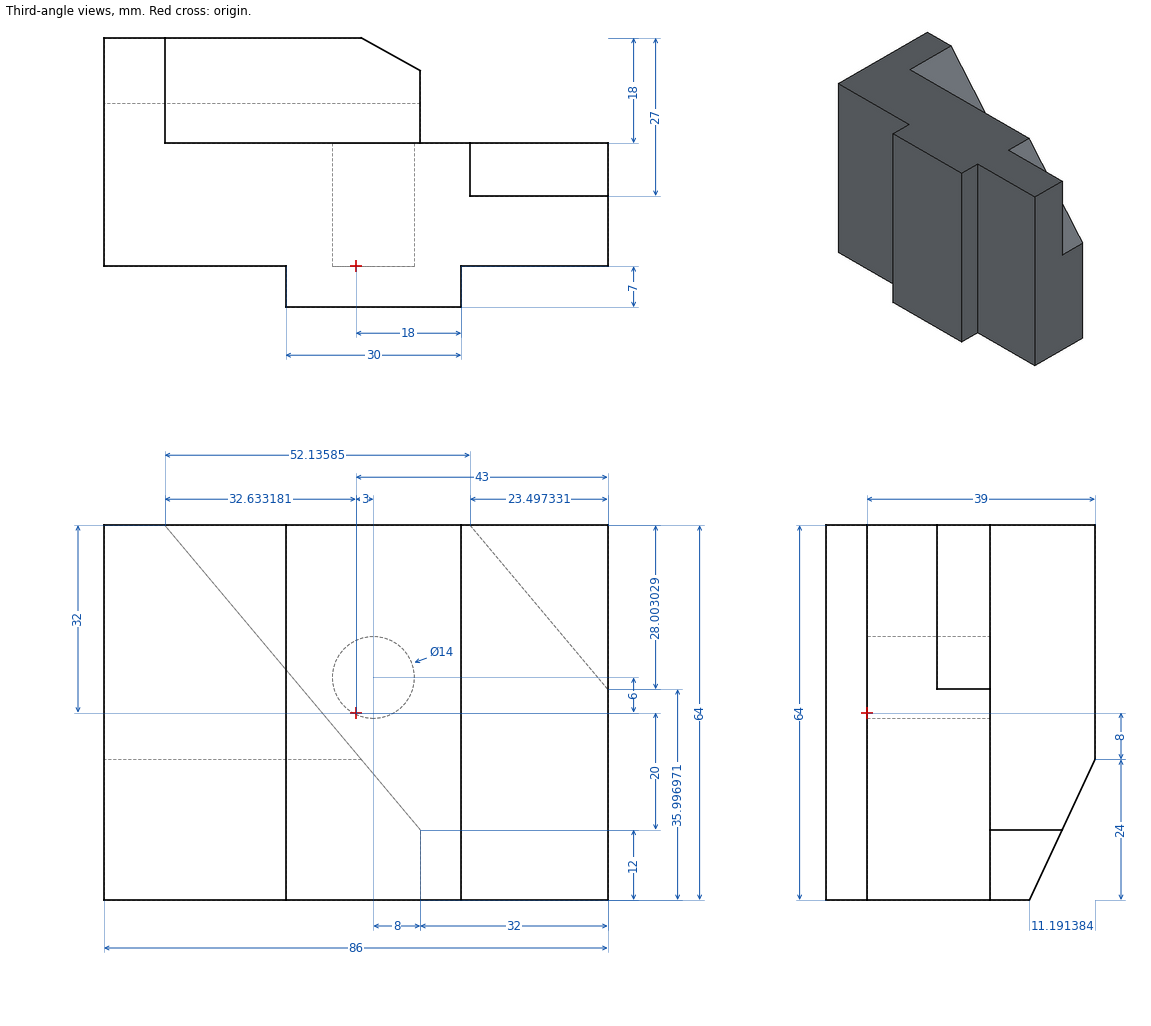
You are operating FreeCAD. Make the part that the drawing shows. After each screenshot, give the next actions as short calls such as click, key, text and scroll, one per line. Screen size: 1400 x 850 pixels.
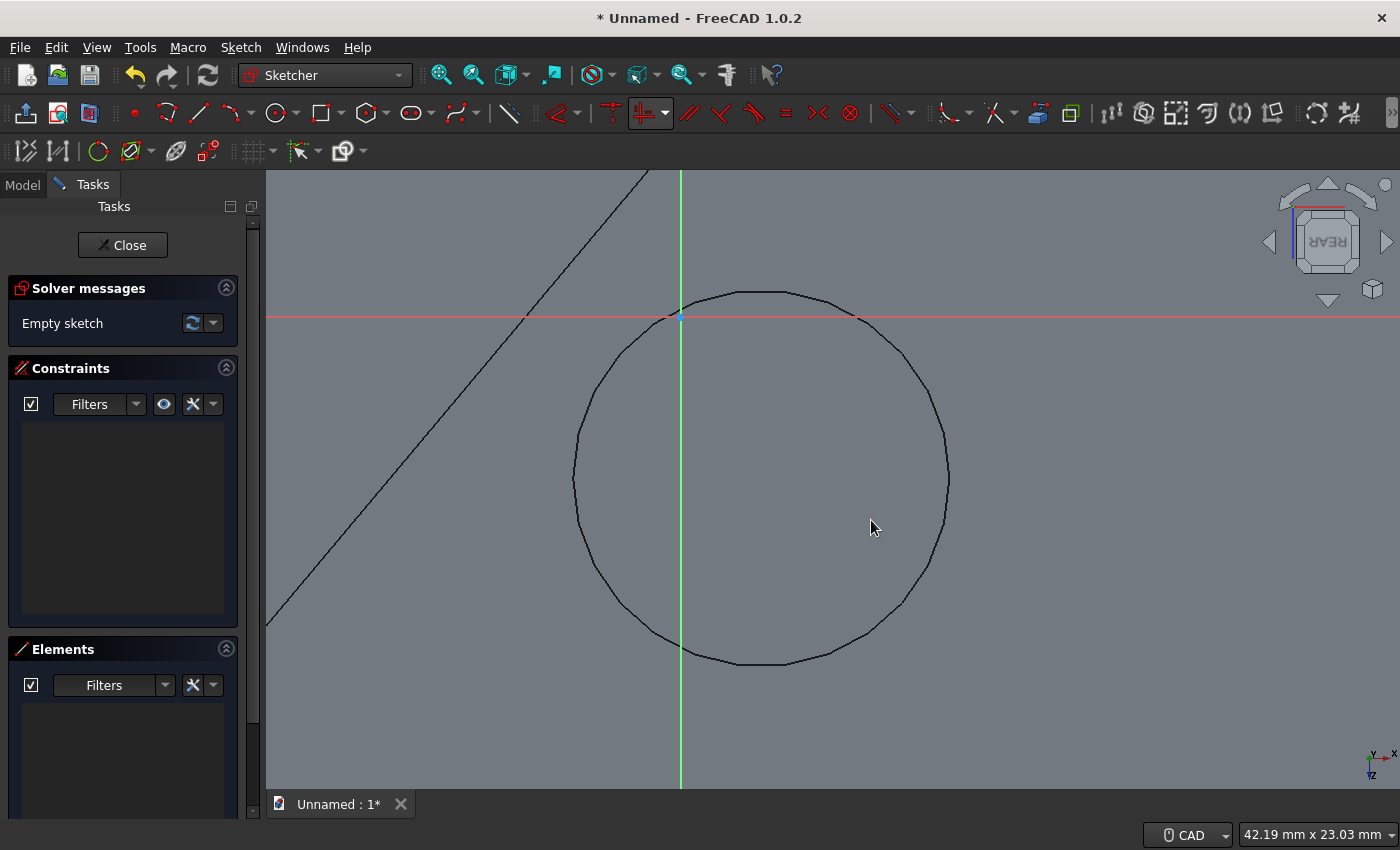
key(g)
key(c)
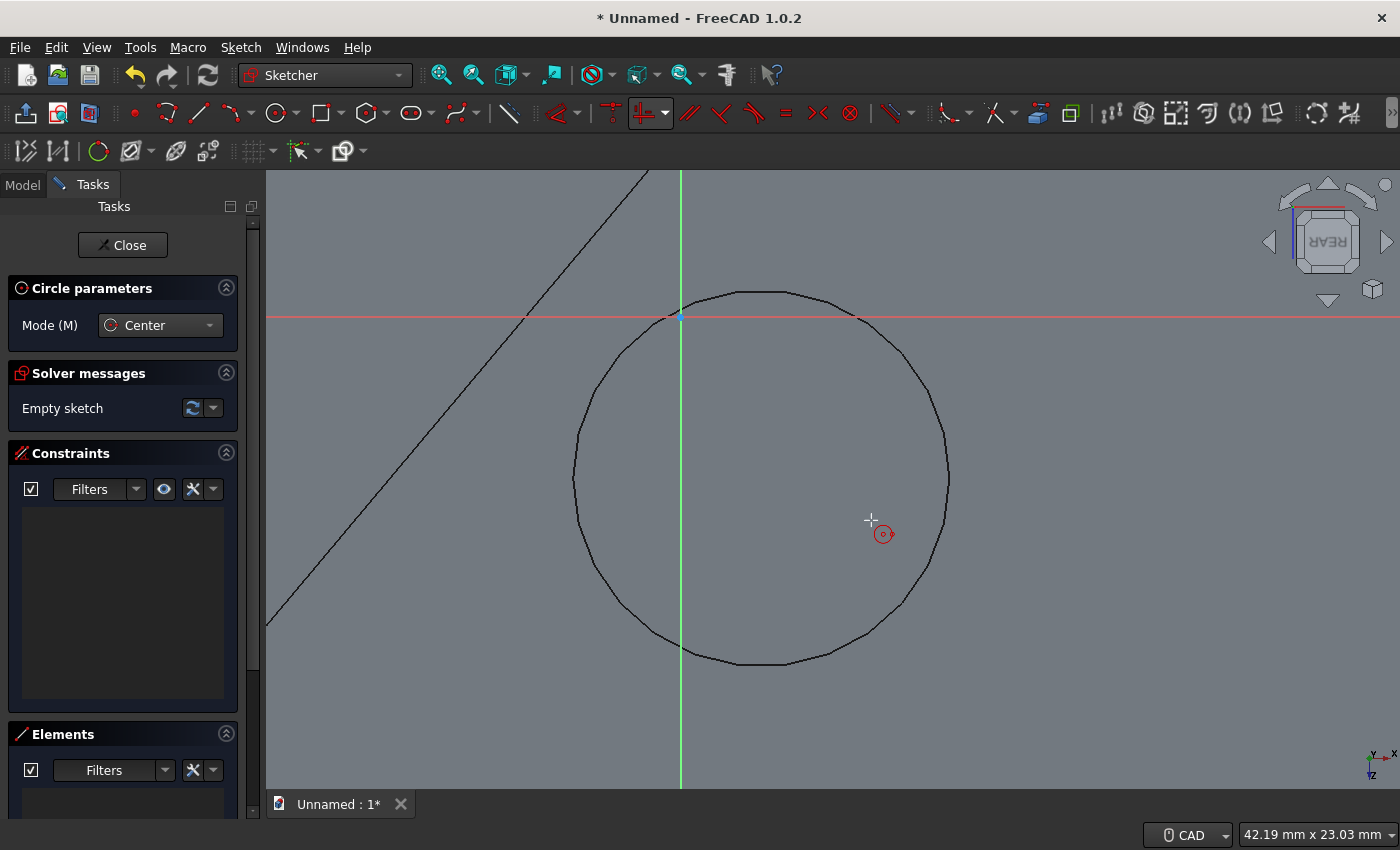
click(761, 478)
move(894, 345)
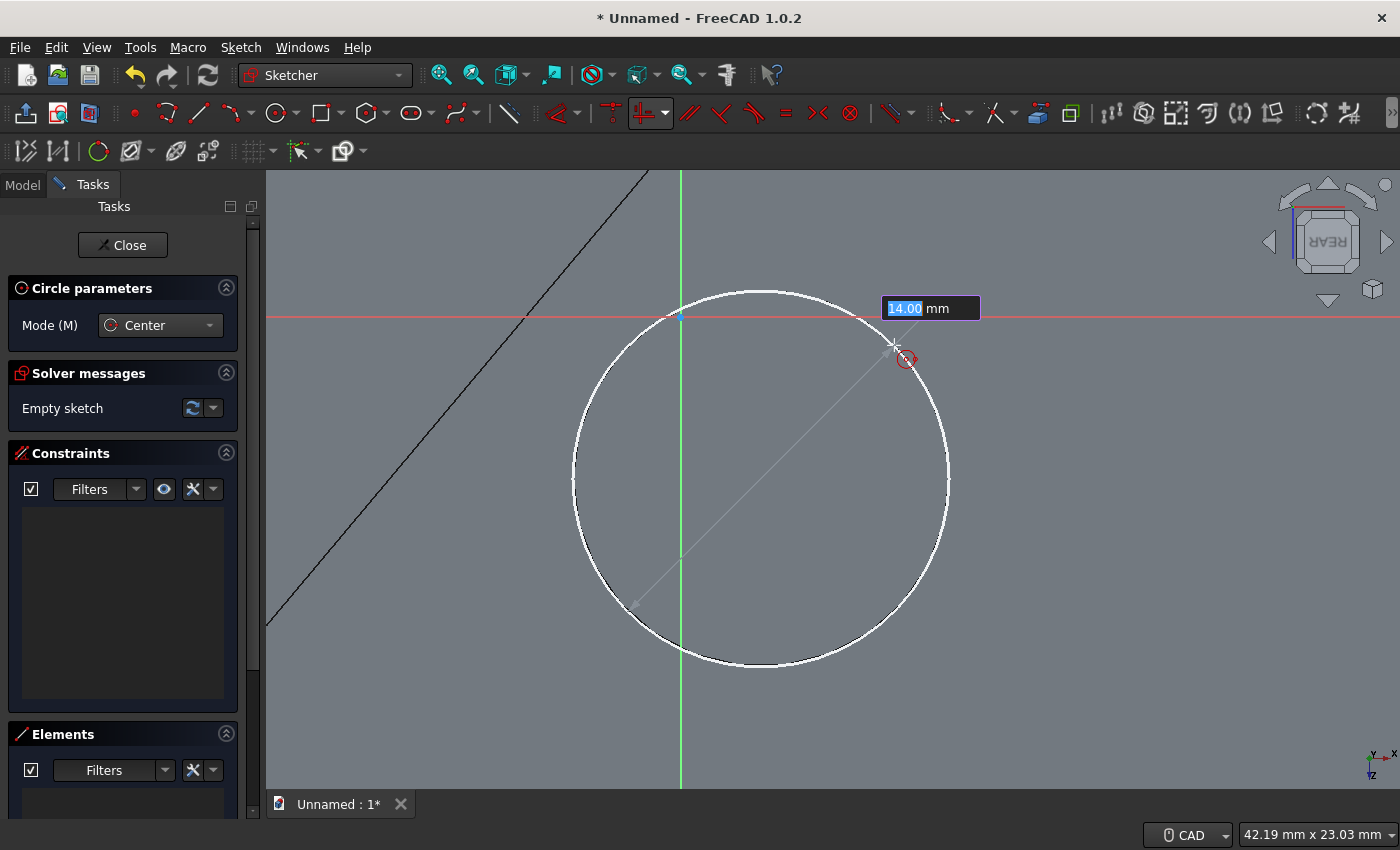
text(14)
key(Return)
key(Escape)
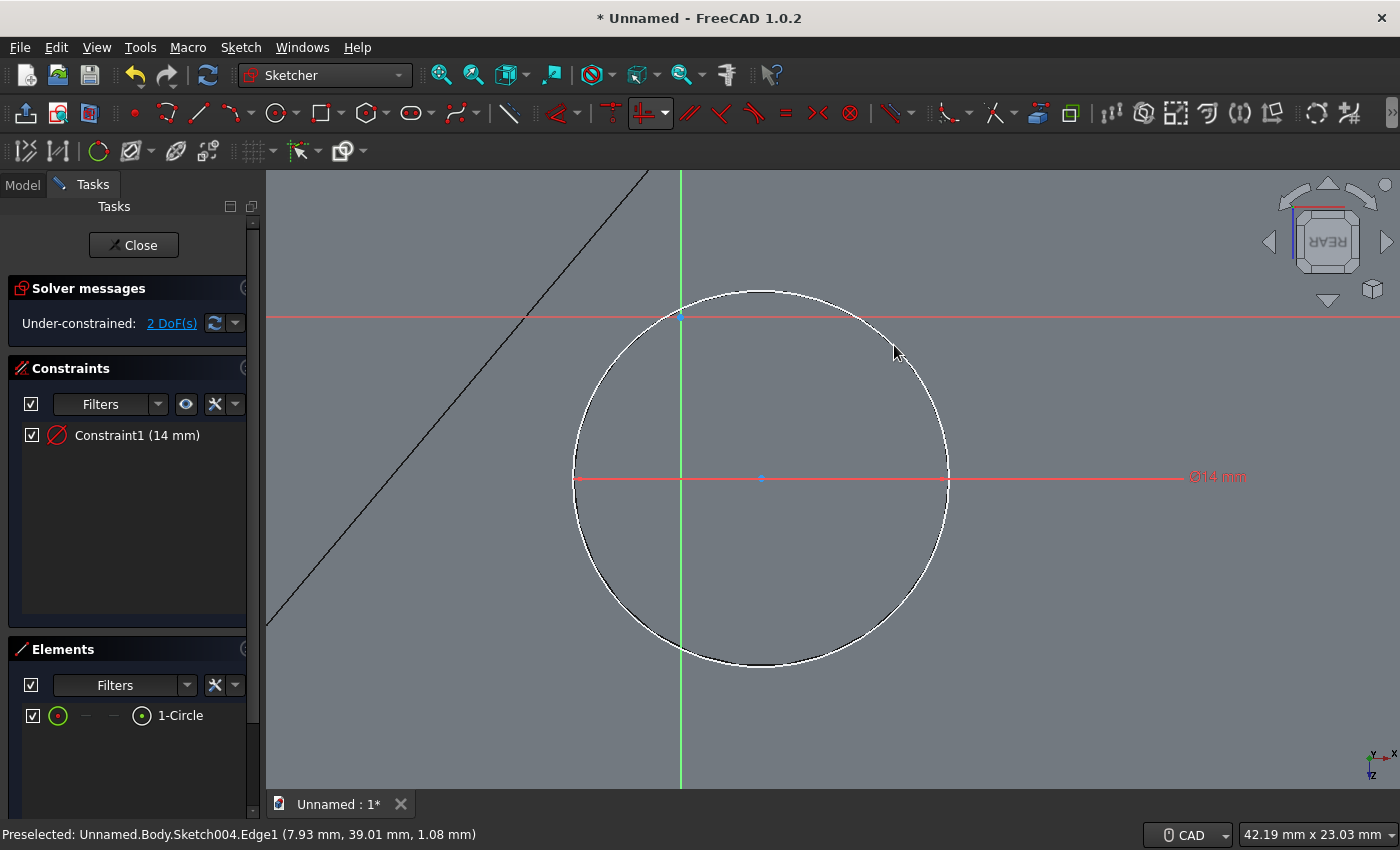
key(d)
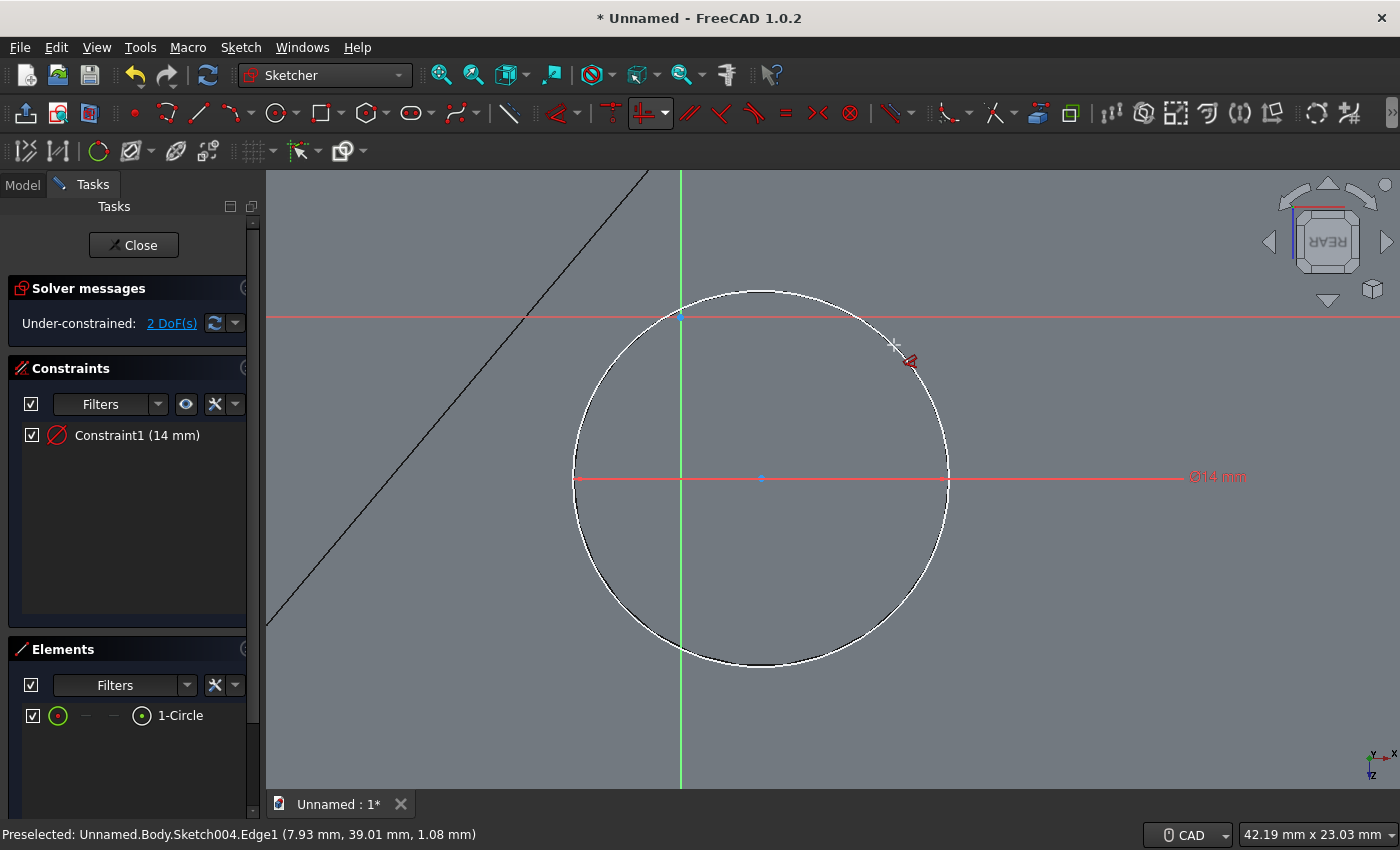
click(761, 479)
click(702, 283)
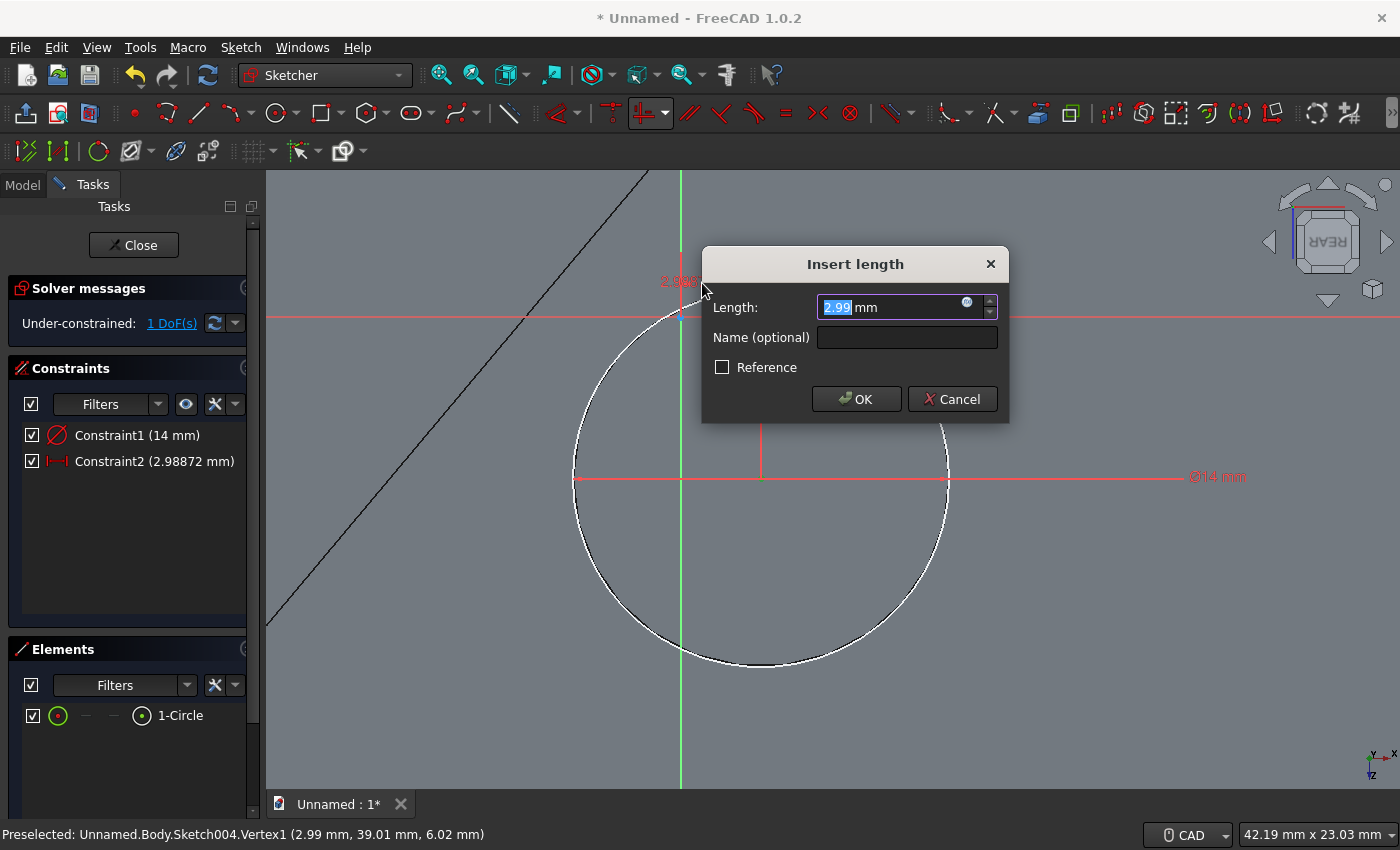
text(3)
key(Return)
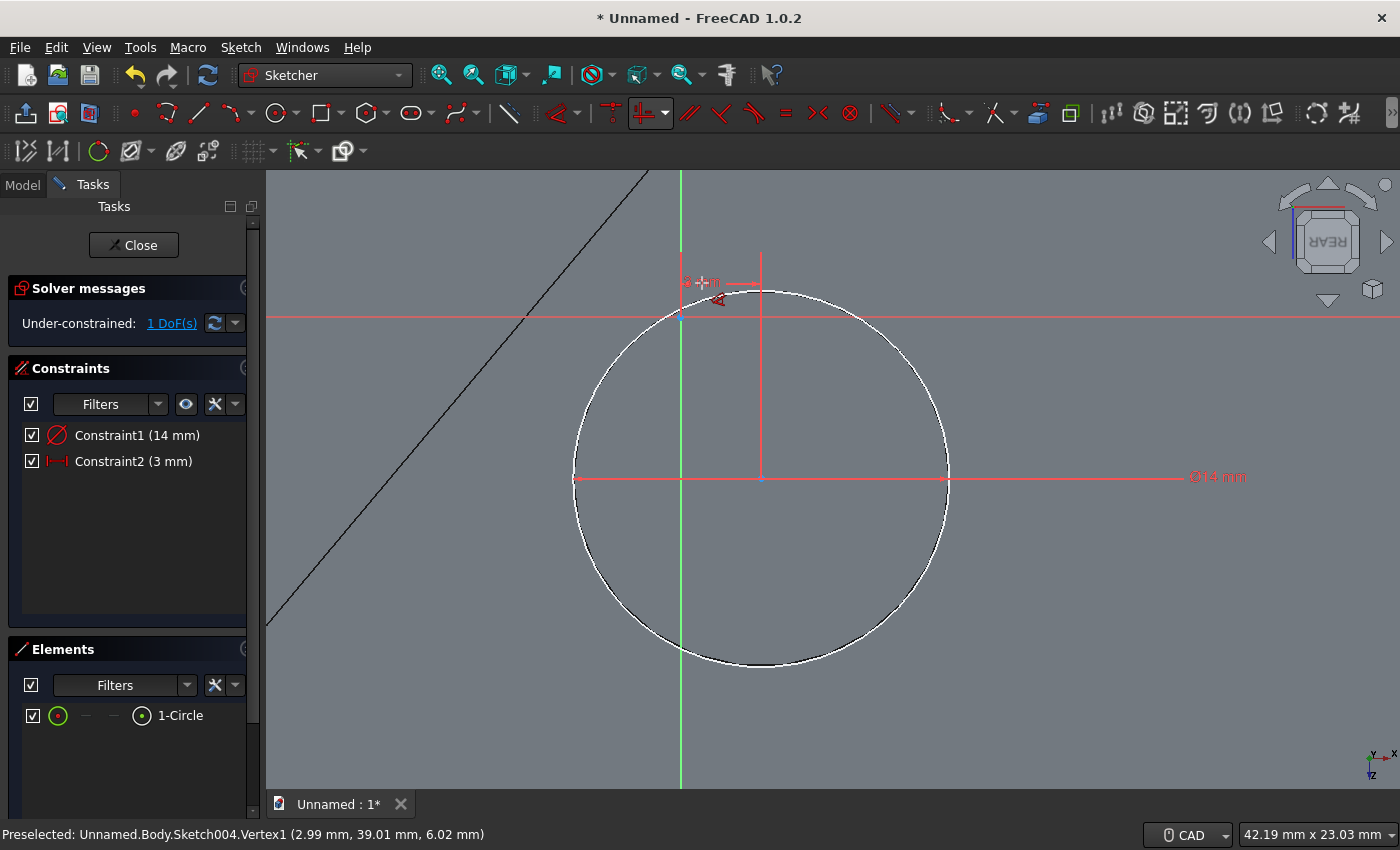
click(761, 479)
click(647, 398)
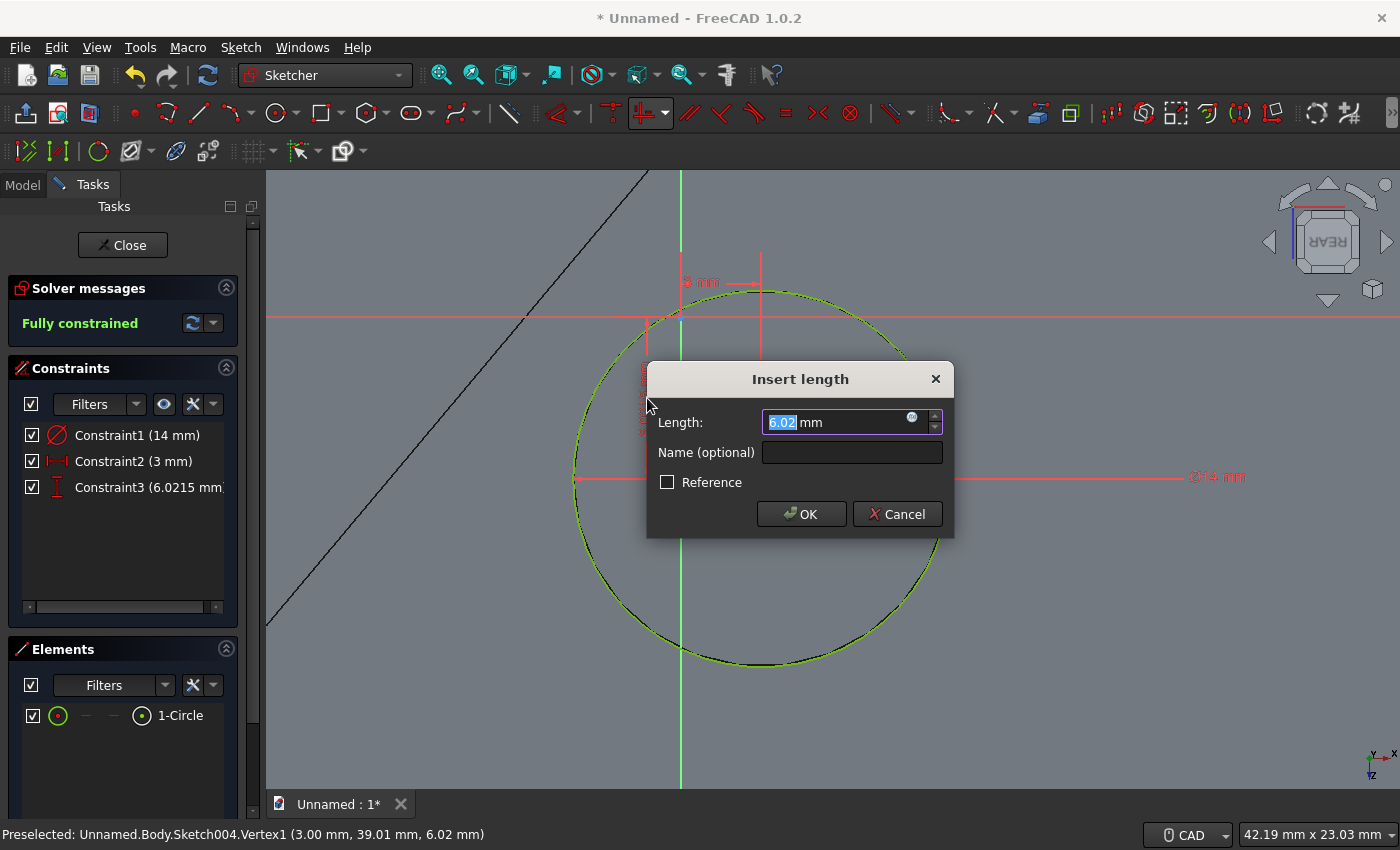
text(6)
key(Return)
key(Escape)